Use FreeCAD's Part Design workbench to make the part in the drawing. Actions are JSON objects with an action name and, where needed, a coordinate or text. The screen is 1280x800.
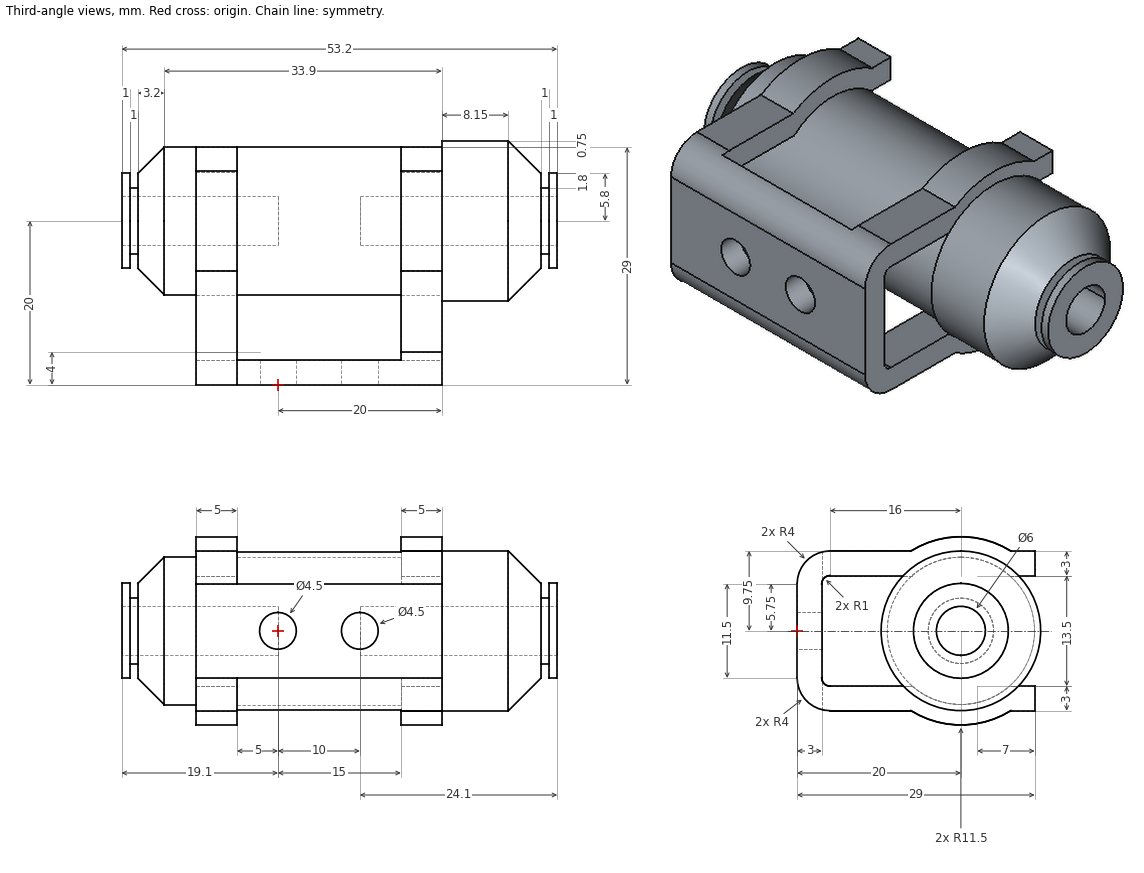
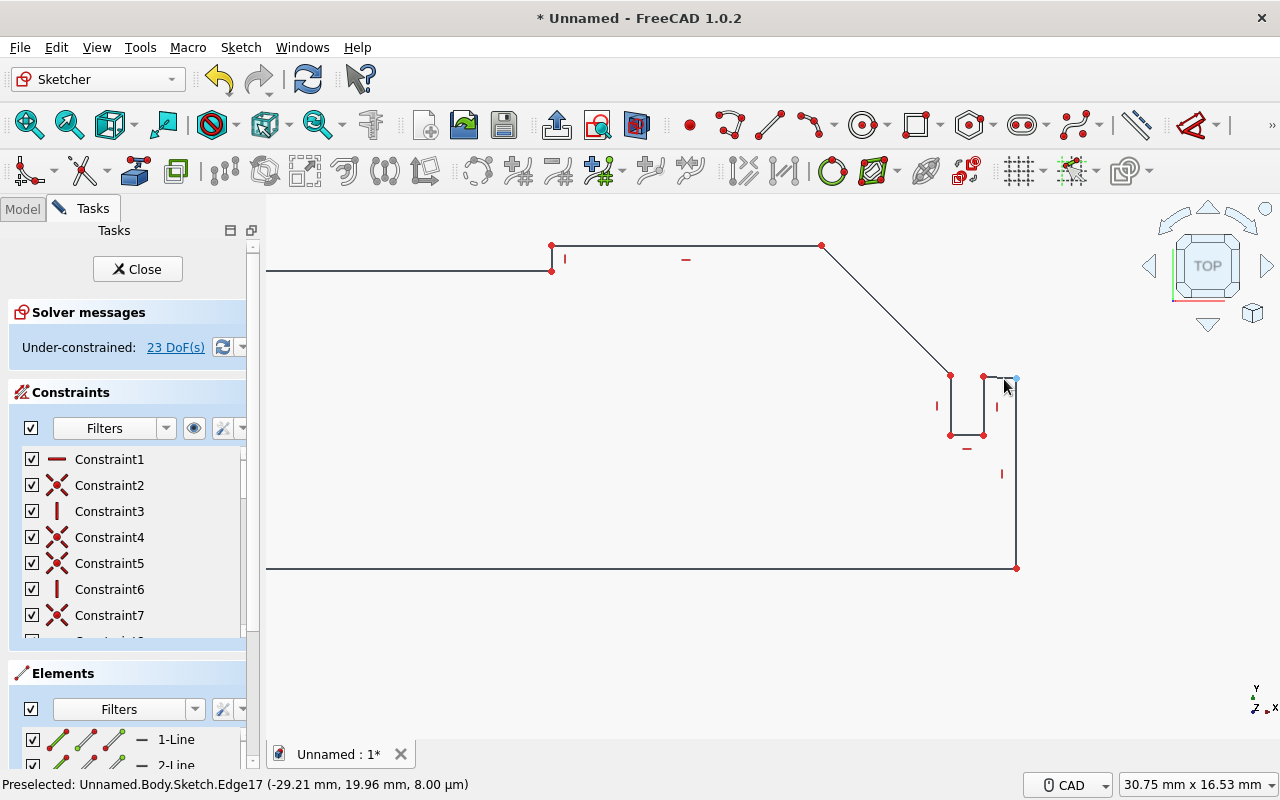
{"action": "left_click", "coordinate": [1000, 378]}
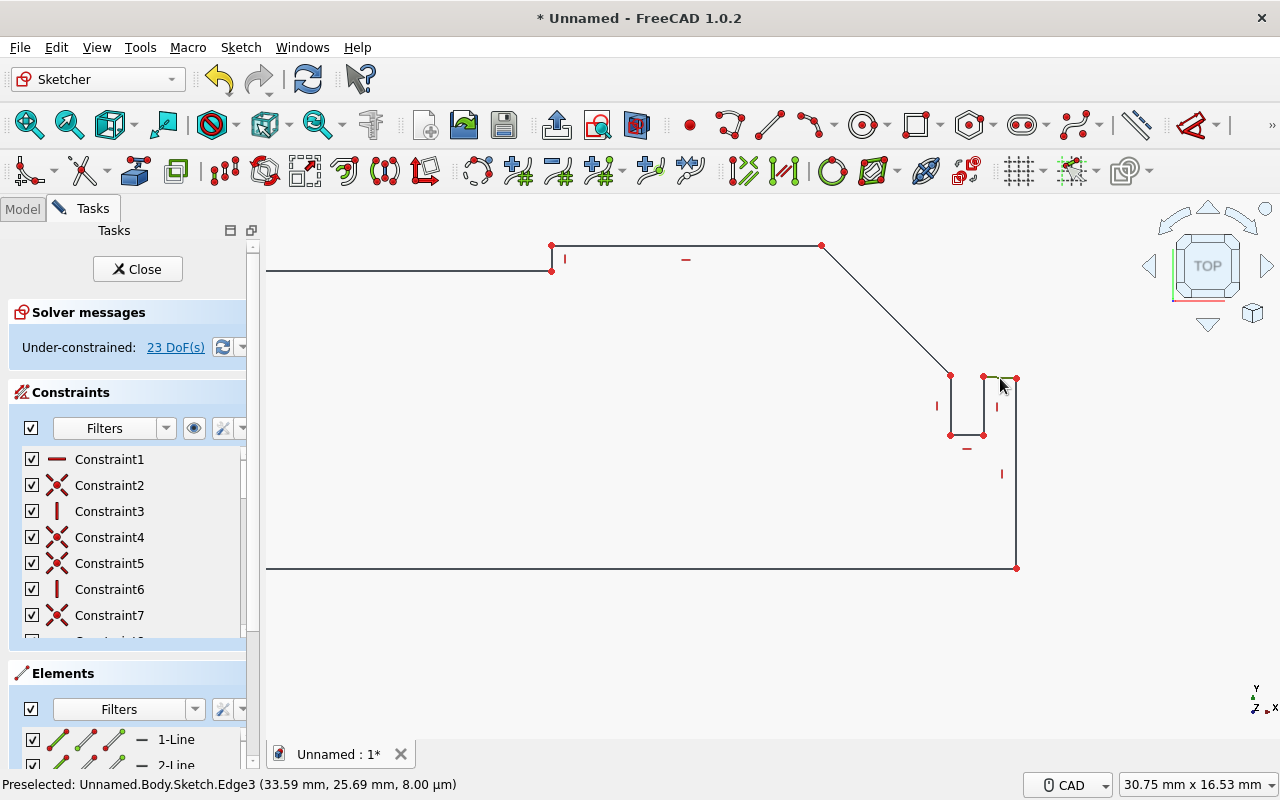
{"action": "key", "text": "h"}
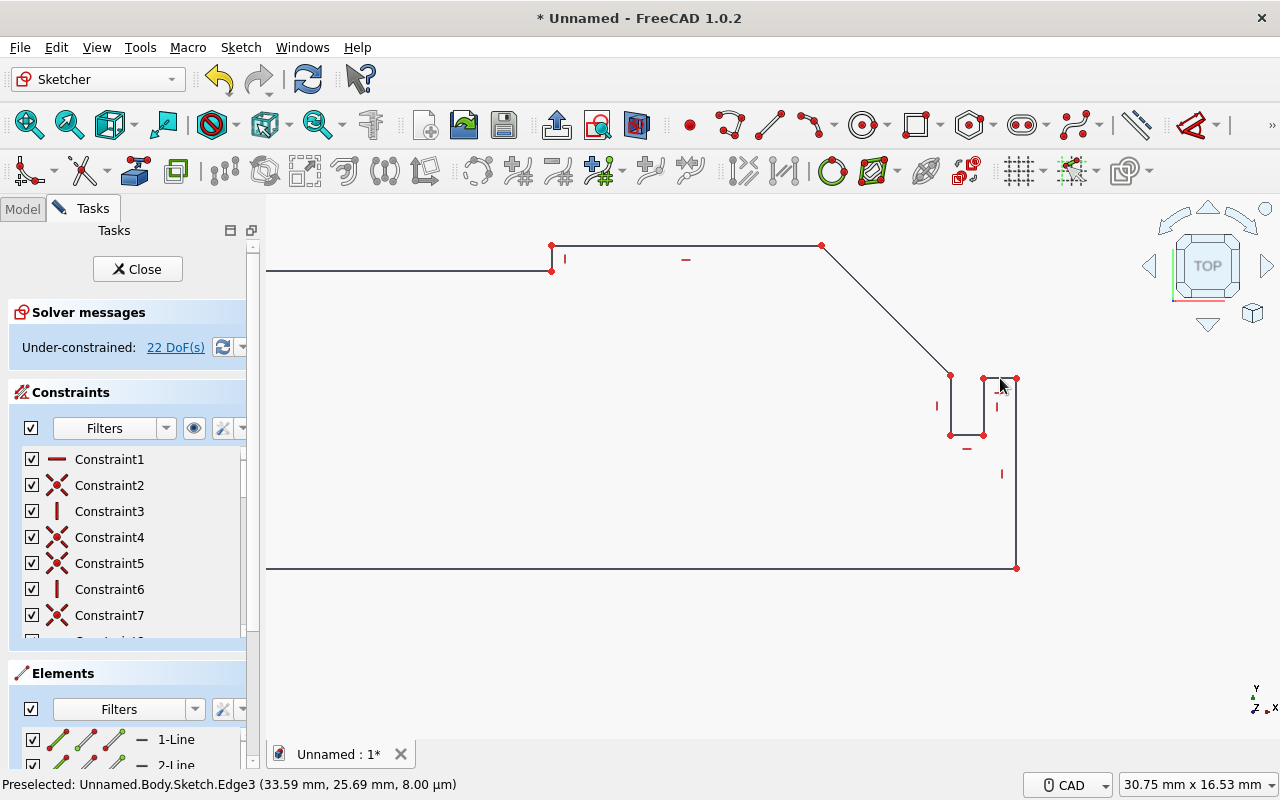
{"action": "scroll", "coordinate": [1004, 379], "scroll_direction": "down", "scroll_amount": 7}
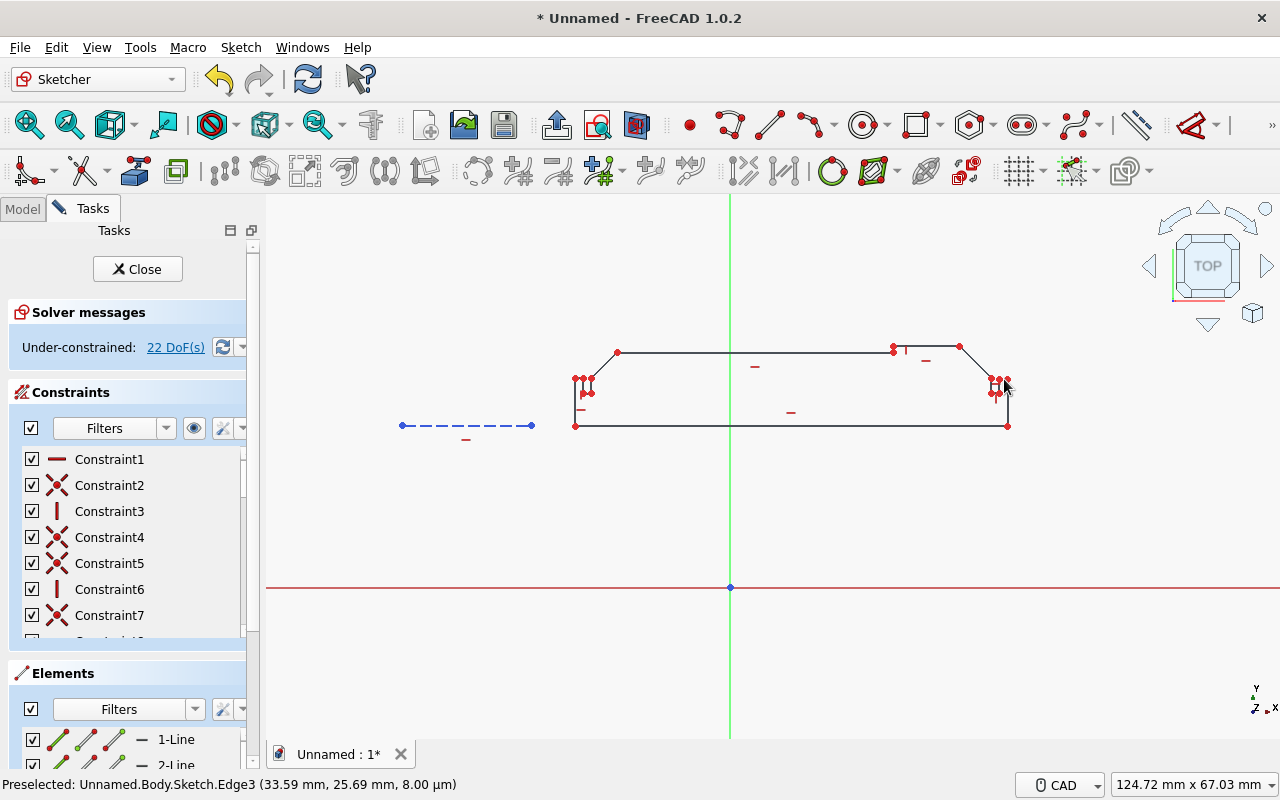
{"action": "scroll", "coordinate": [589, 394], "scroll_direction": "up", "scroll_amount": 9}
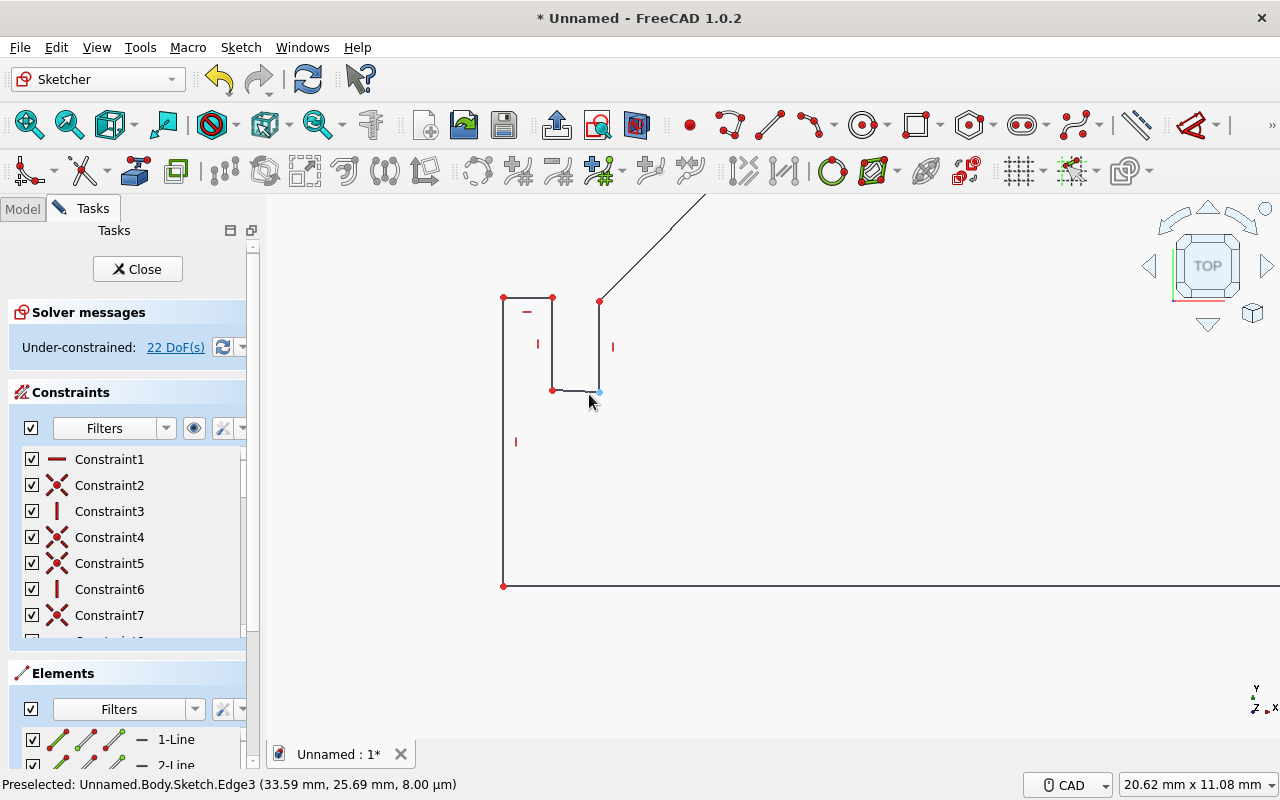
{"action": "left_click", "coordinate": [585, 392]}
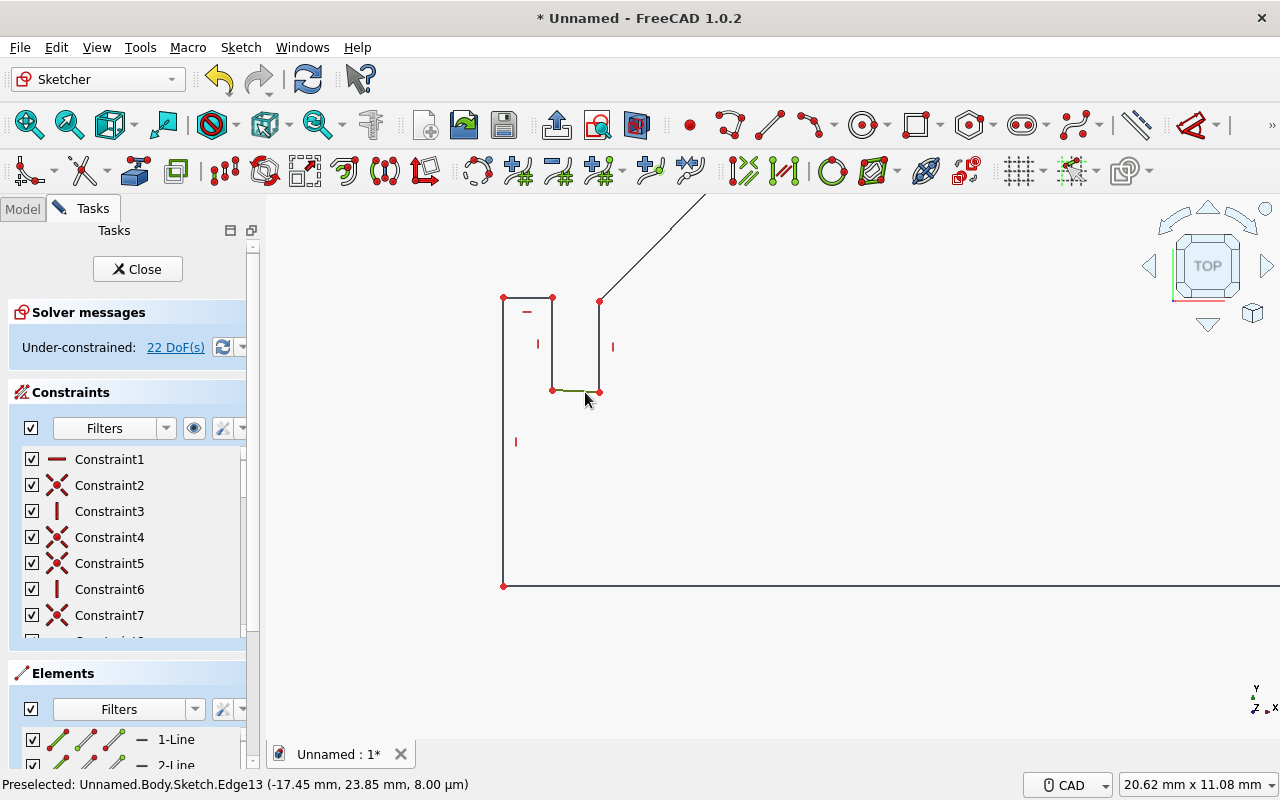
{"action": "key", "text": "h"}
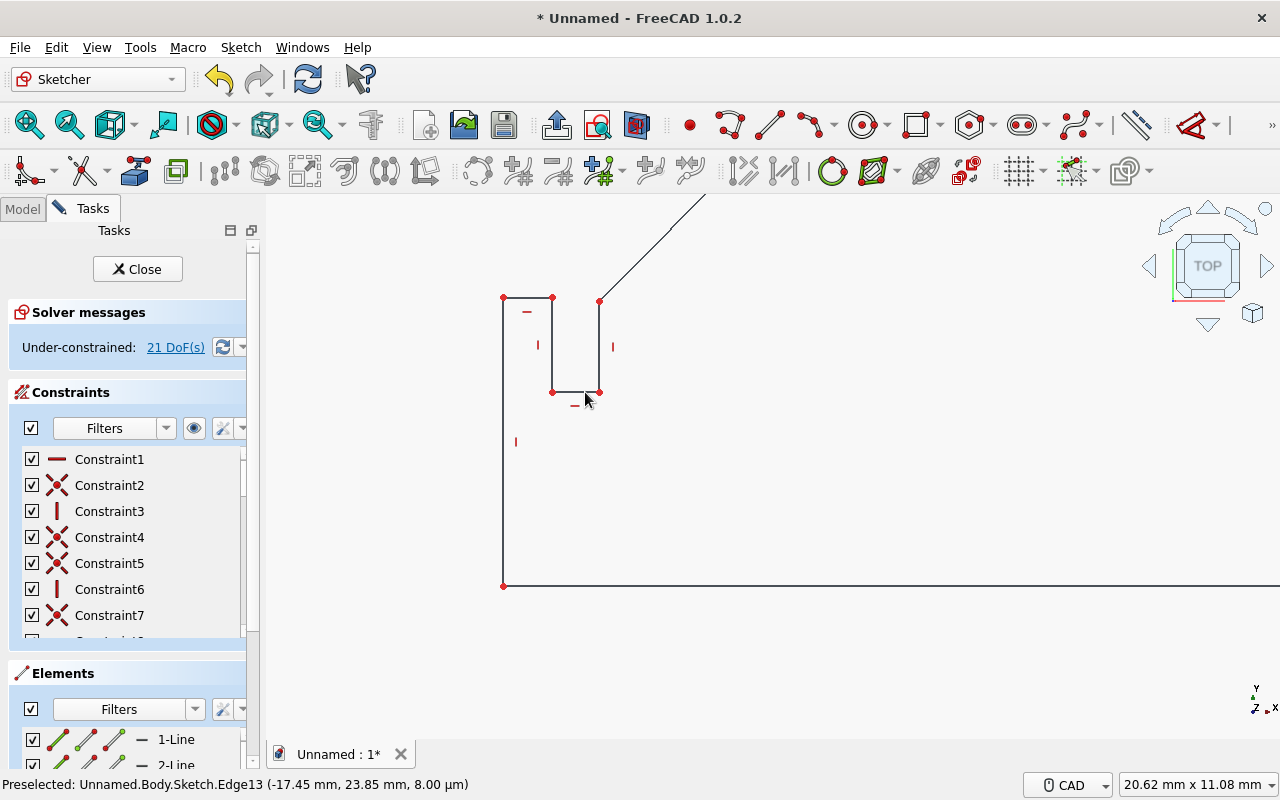
{"action": "scroll", "coordinate": [589, 394], "scroll_direction": "down", "scroll_amount": 9}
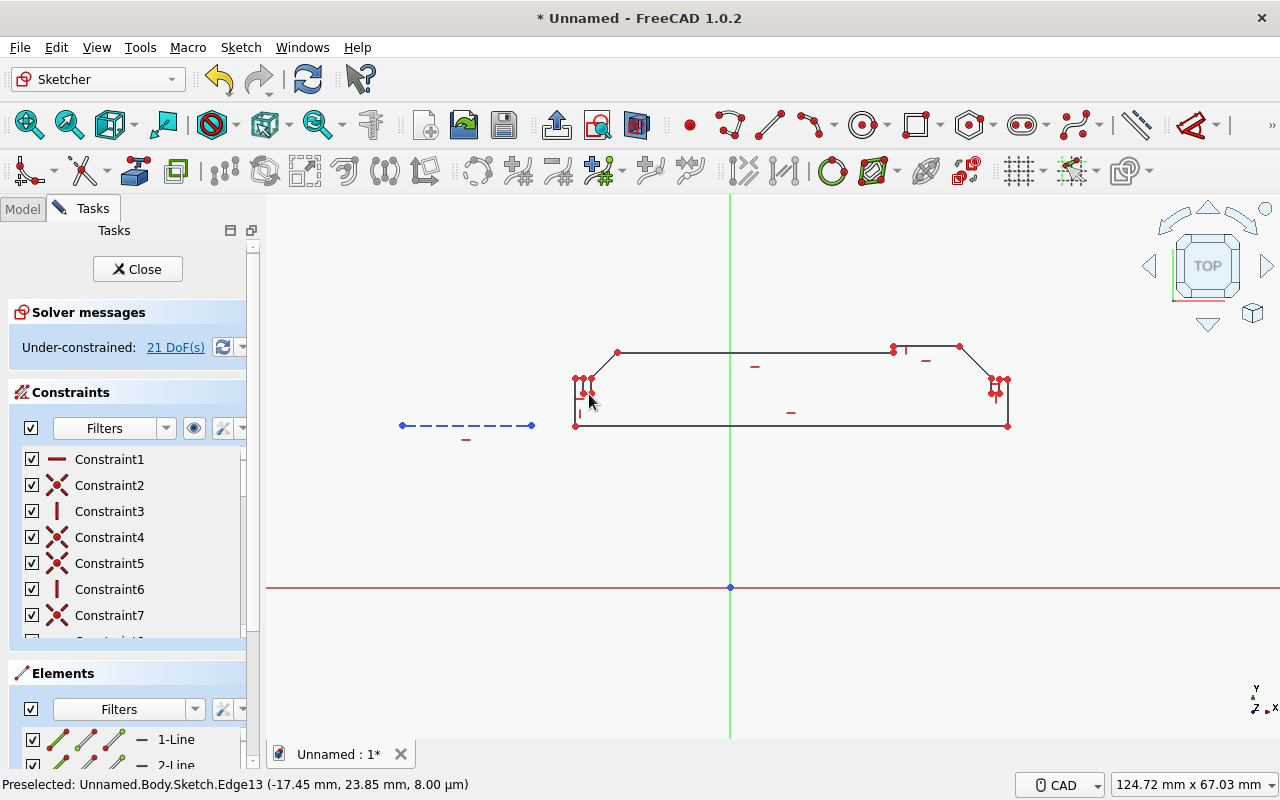
{"action": "scroll", "coordinate": [1005, 379], "scroll_direction": "up", "scroll_amount": 9}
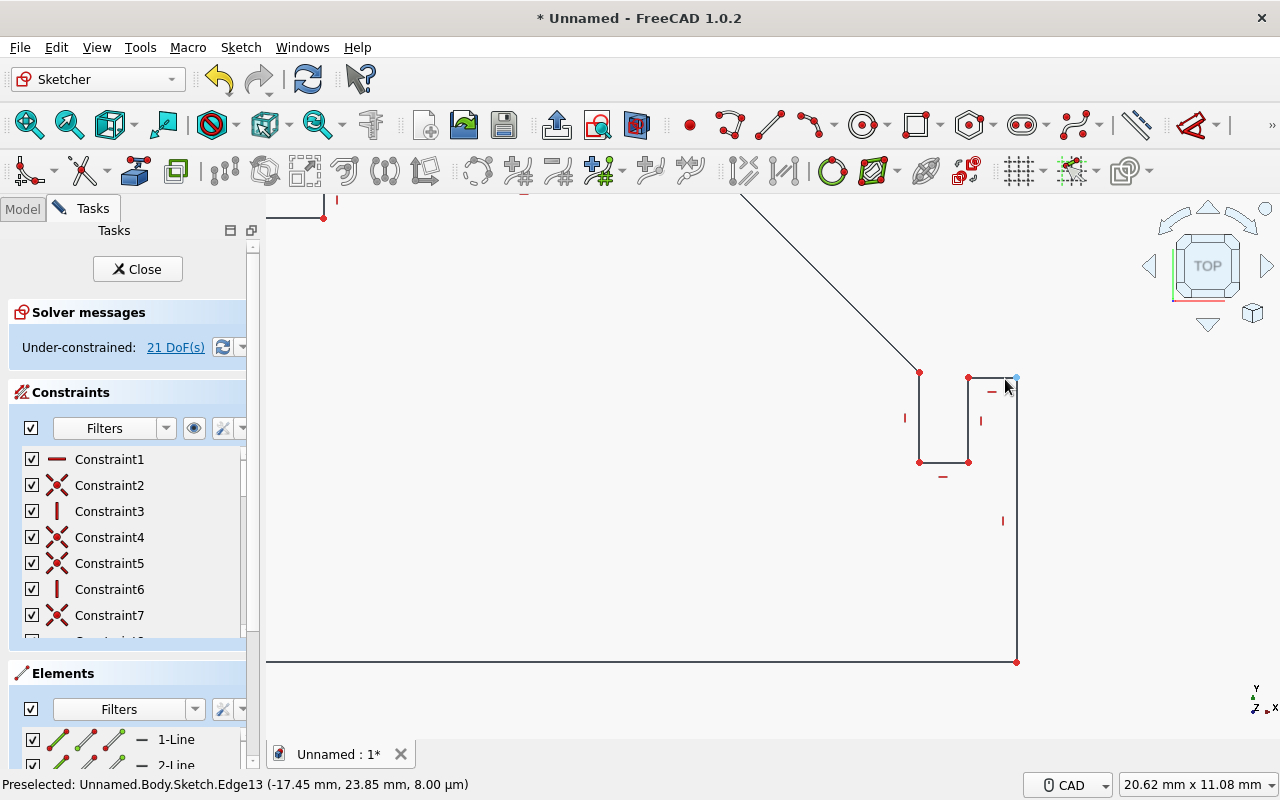
{"action": "left_click", "coordinate": [1002, 378]}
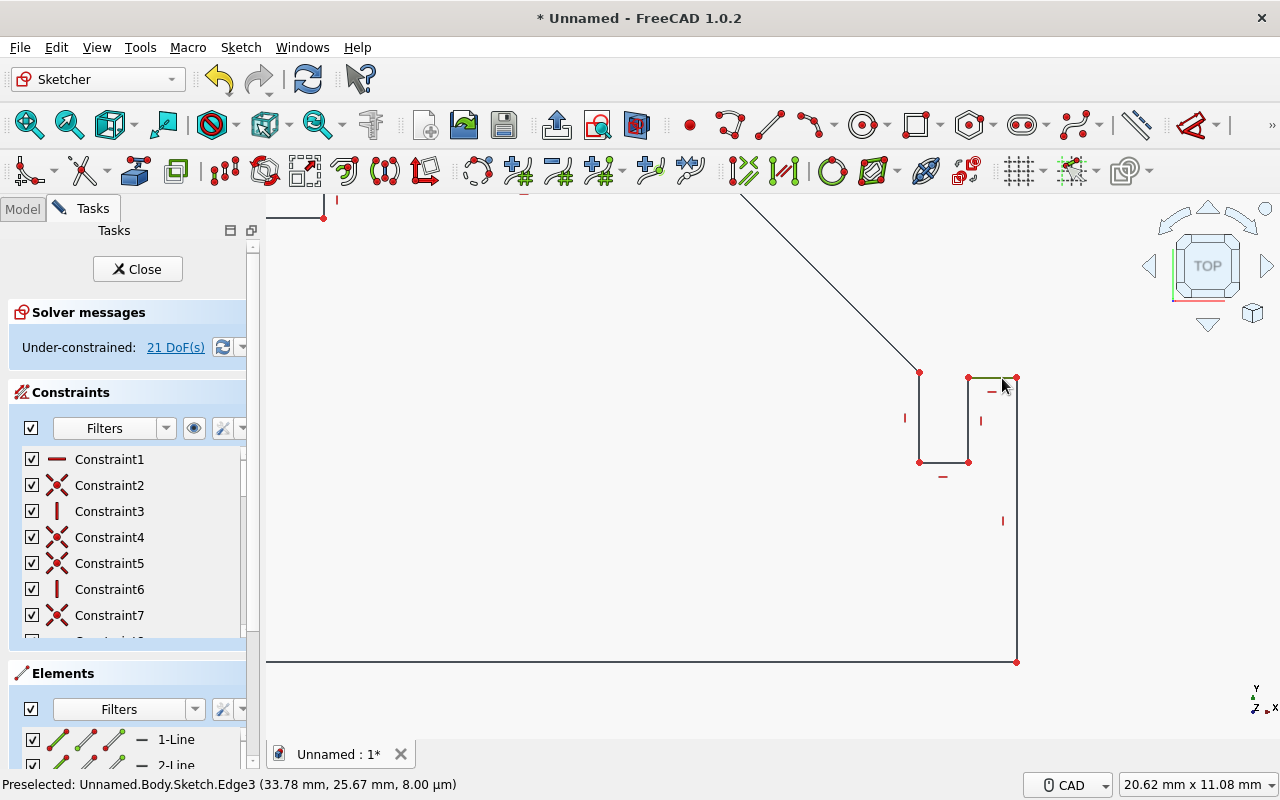
{"action": "left_click", "coordinate": [1218, 126]}